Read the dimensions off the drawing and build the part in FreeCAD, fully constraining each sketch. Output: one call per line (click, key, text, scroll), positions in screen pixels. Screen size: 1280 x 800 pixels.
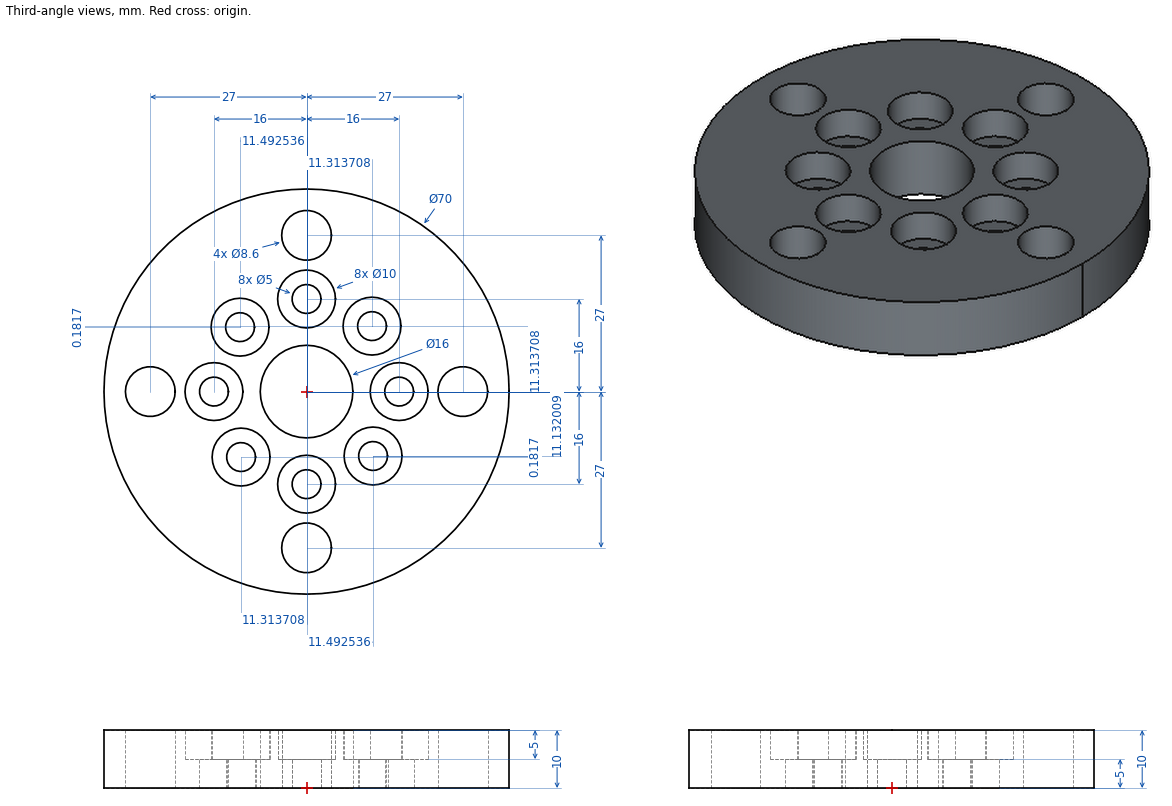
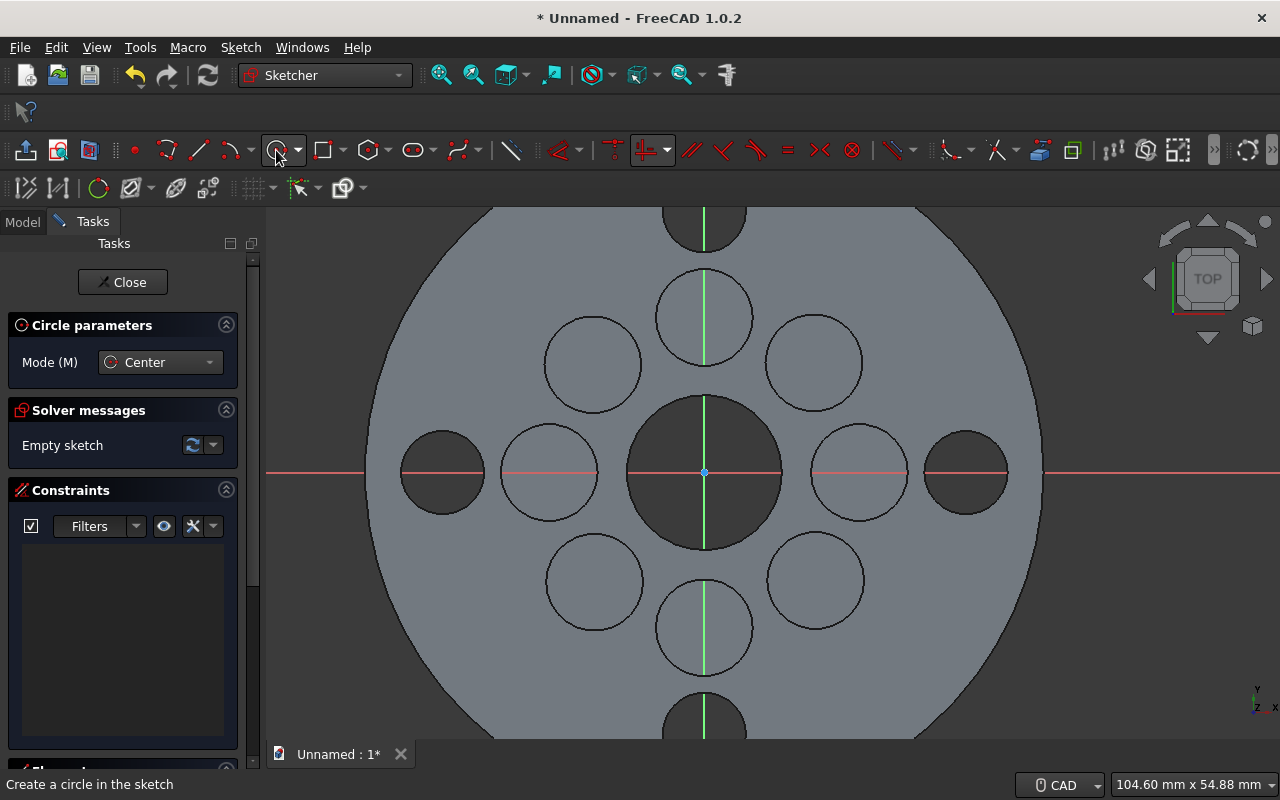
click(704, 317)
move(721, 300)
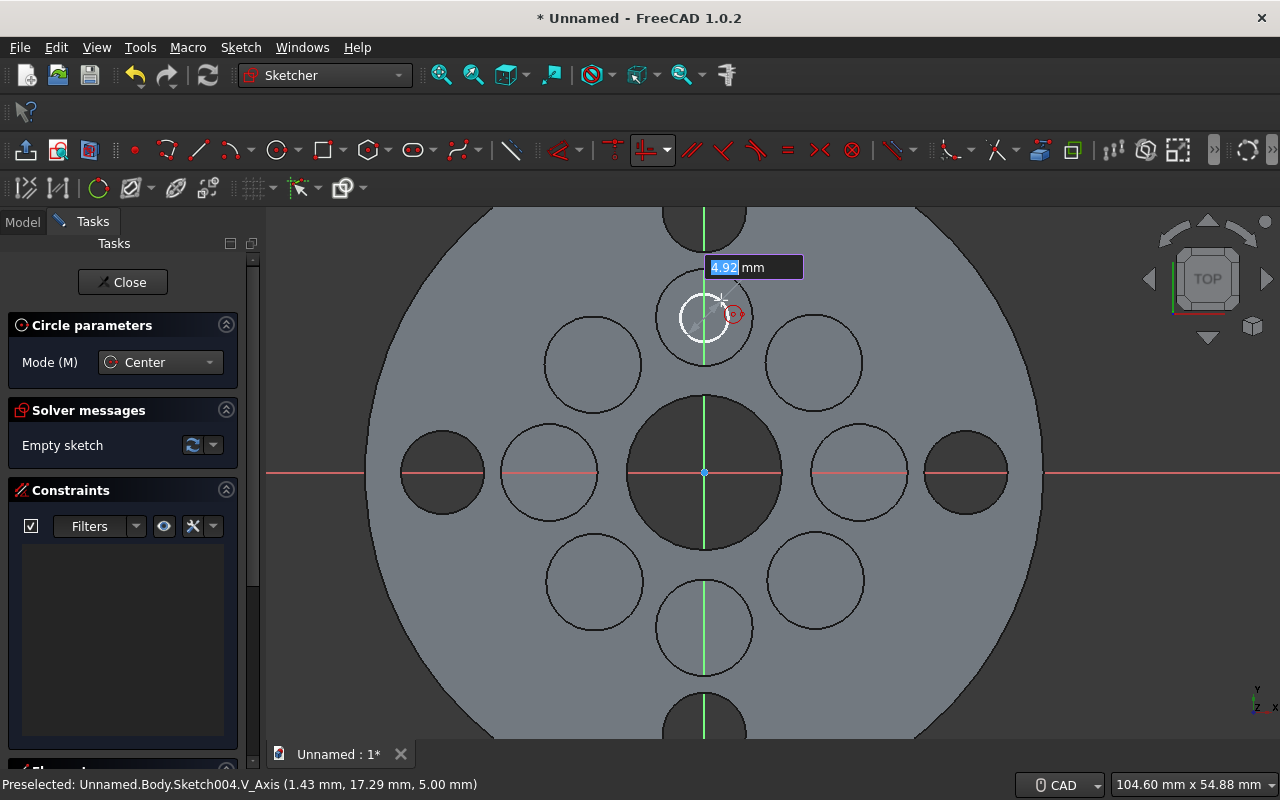
text(5)
key(Return)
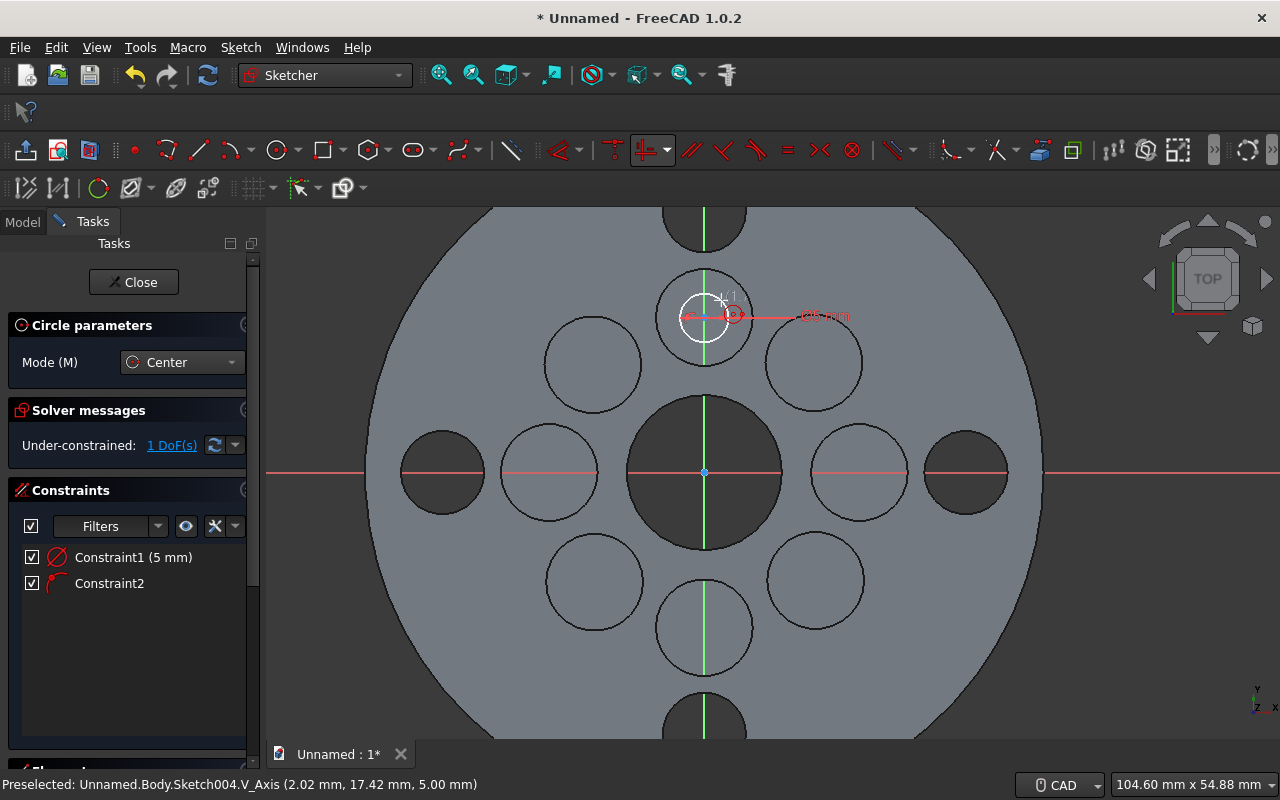
click(814, 363)
move(831, 346)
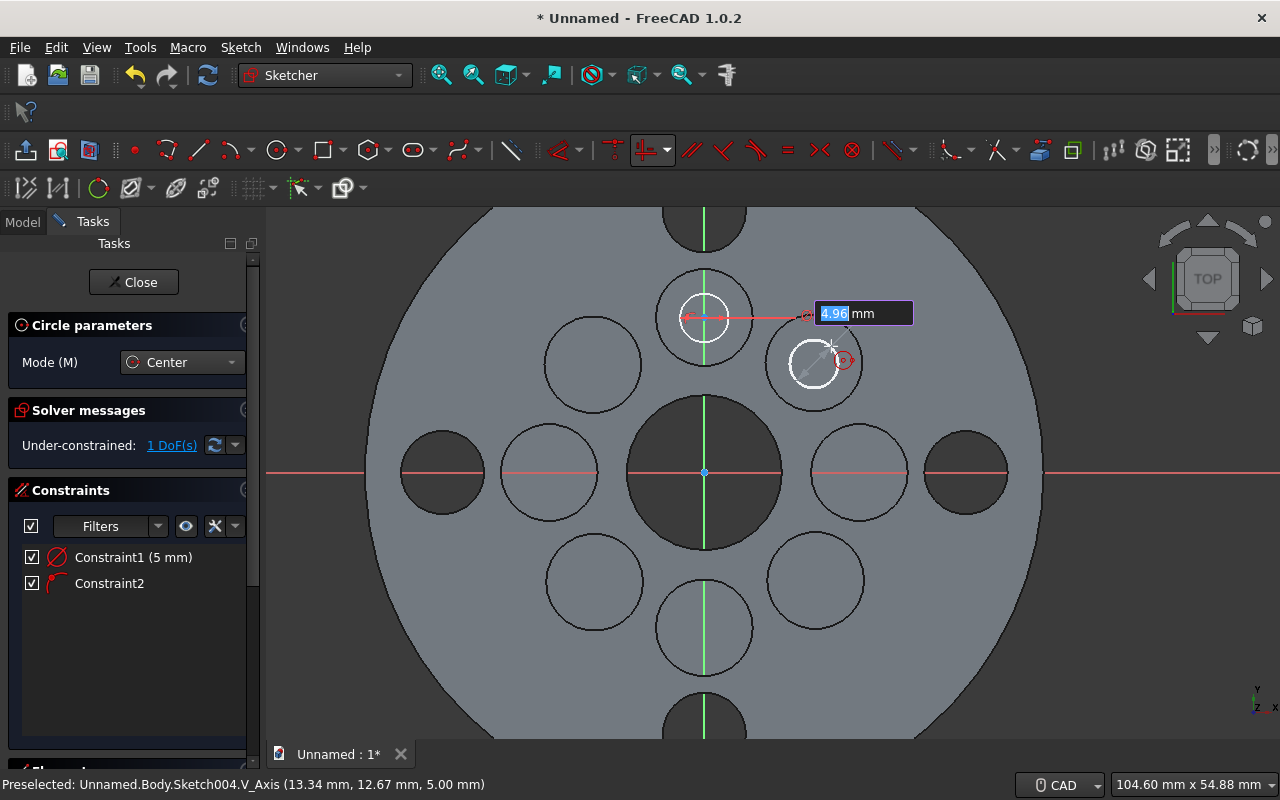
text(5)
key(Return)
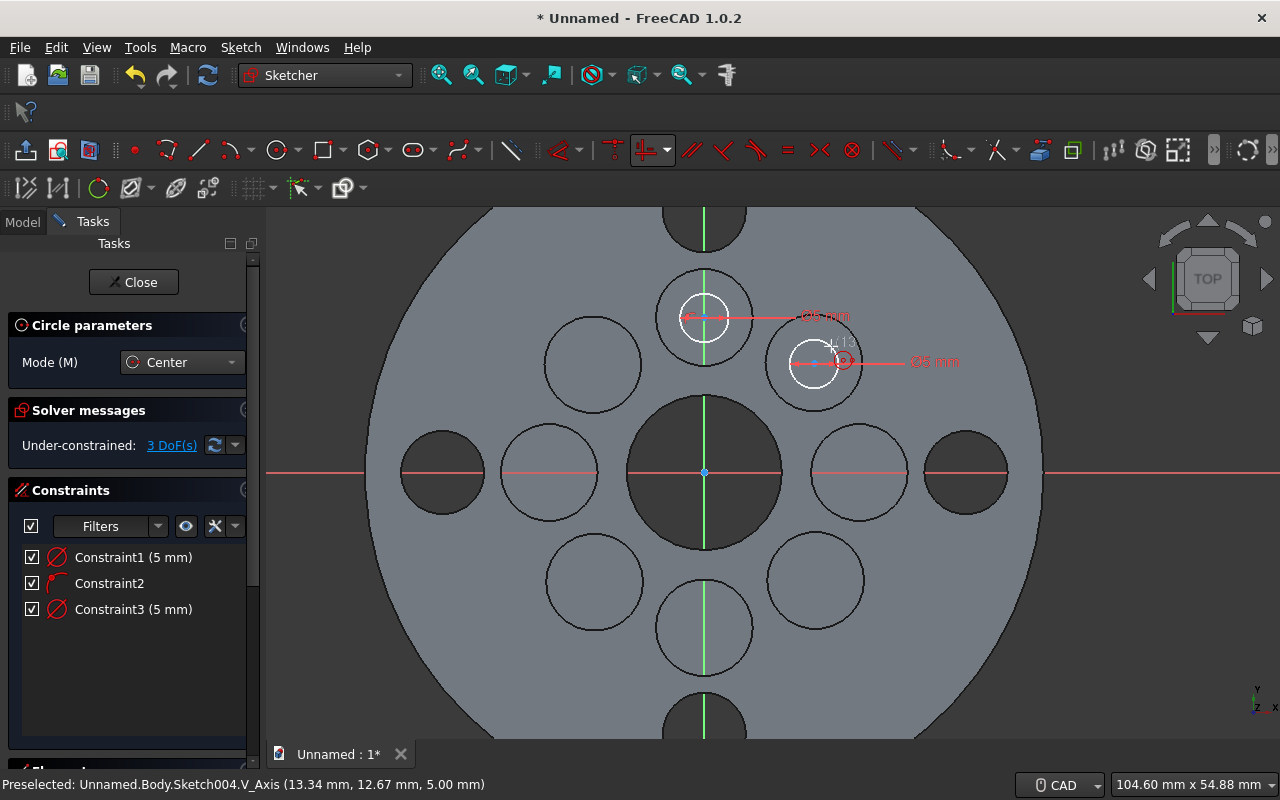
click(859, 473)
move(877, 455)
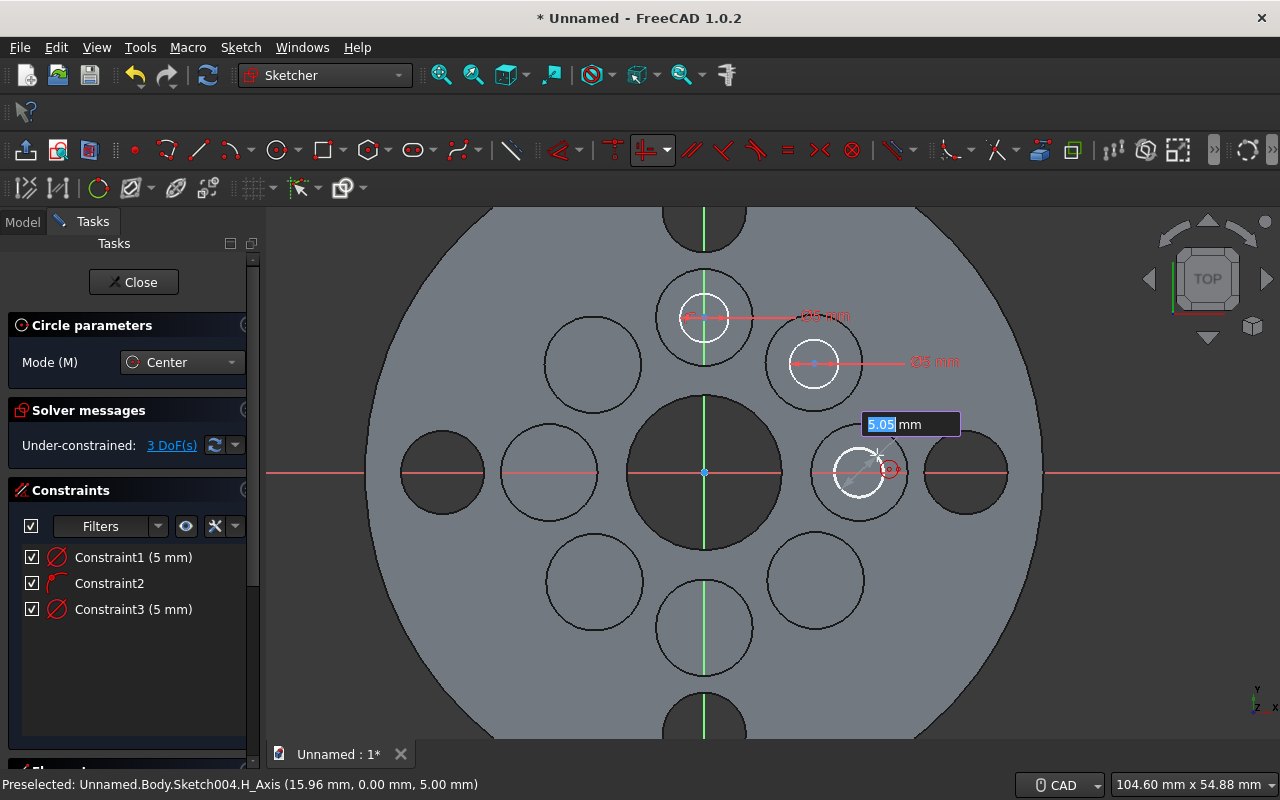
text(5)
key(Return)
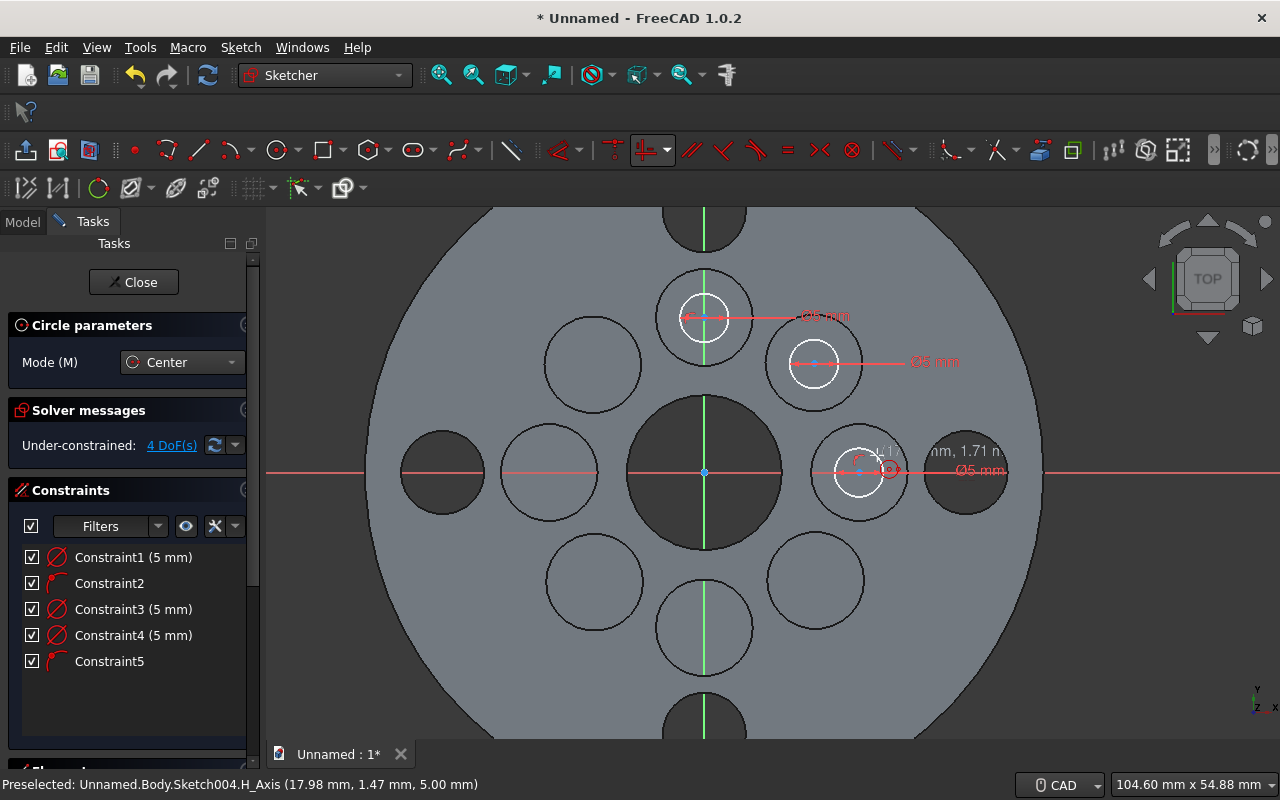
click(816, 580)
move(833, 563)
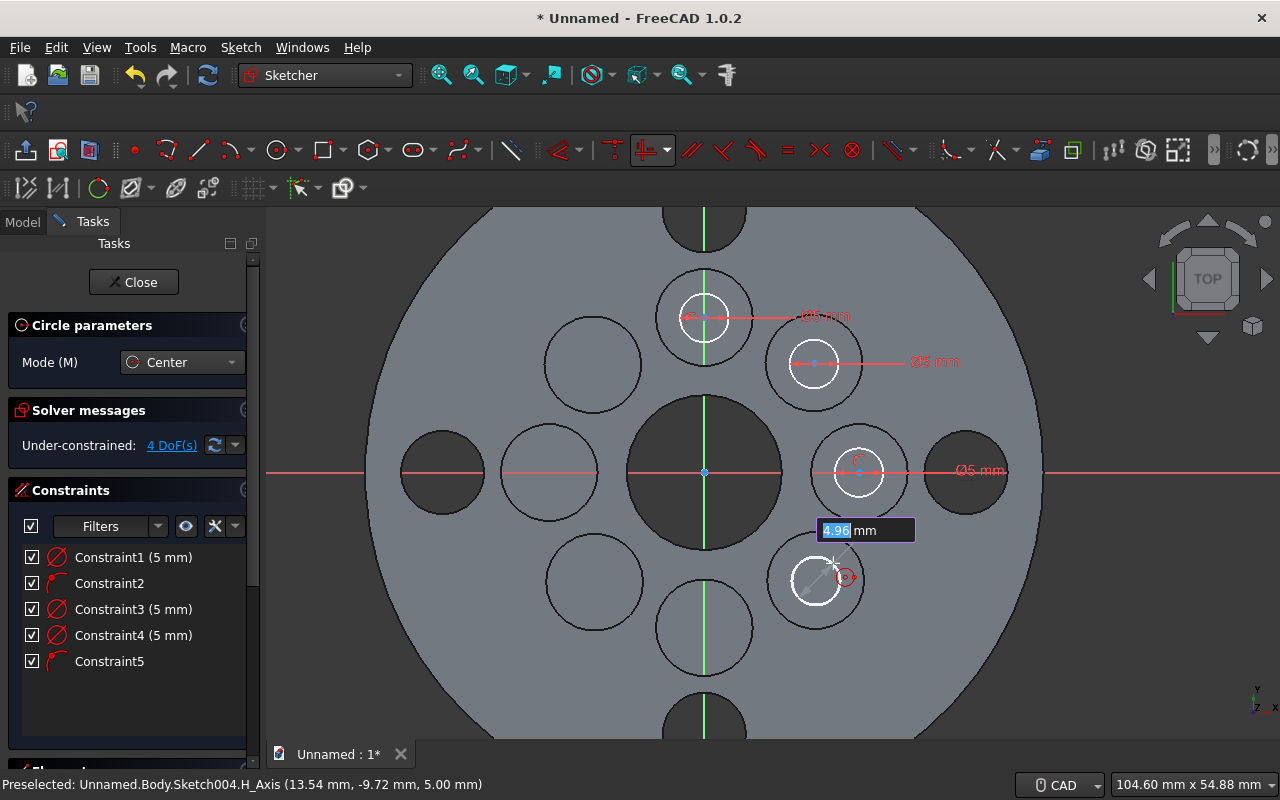
text(5)
key(Return)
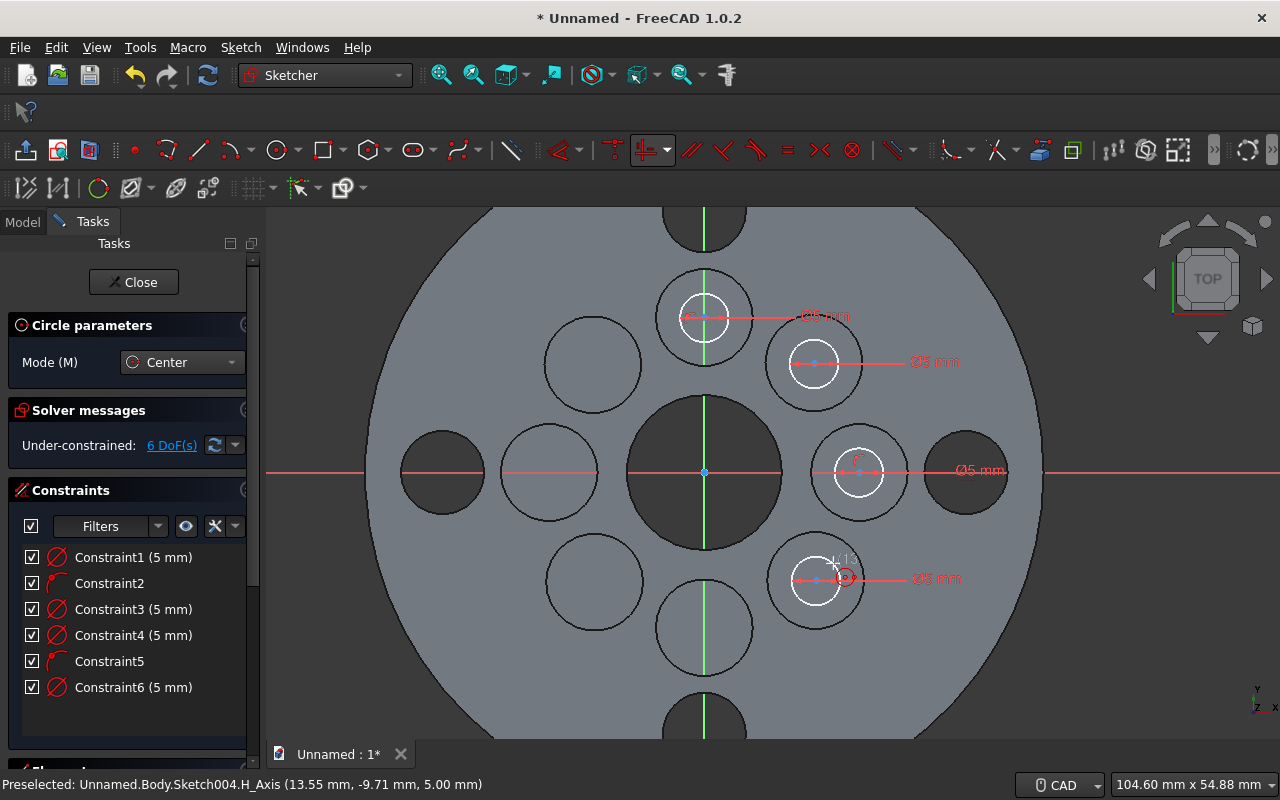
click(704, 628)
move(721, 611)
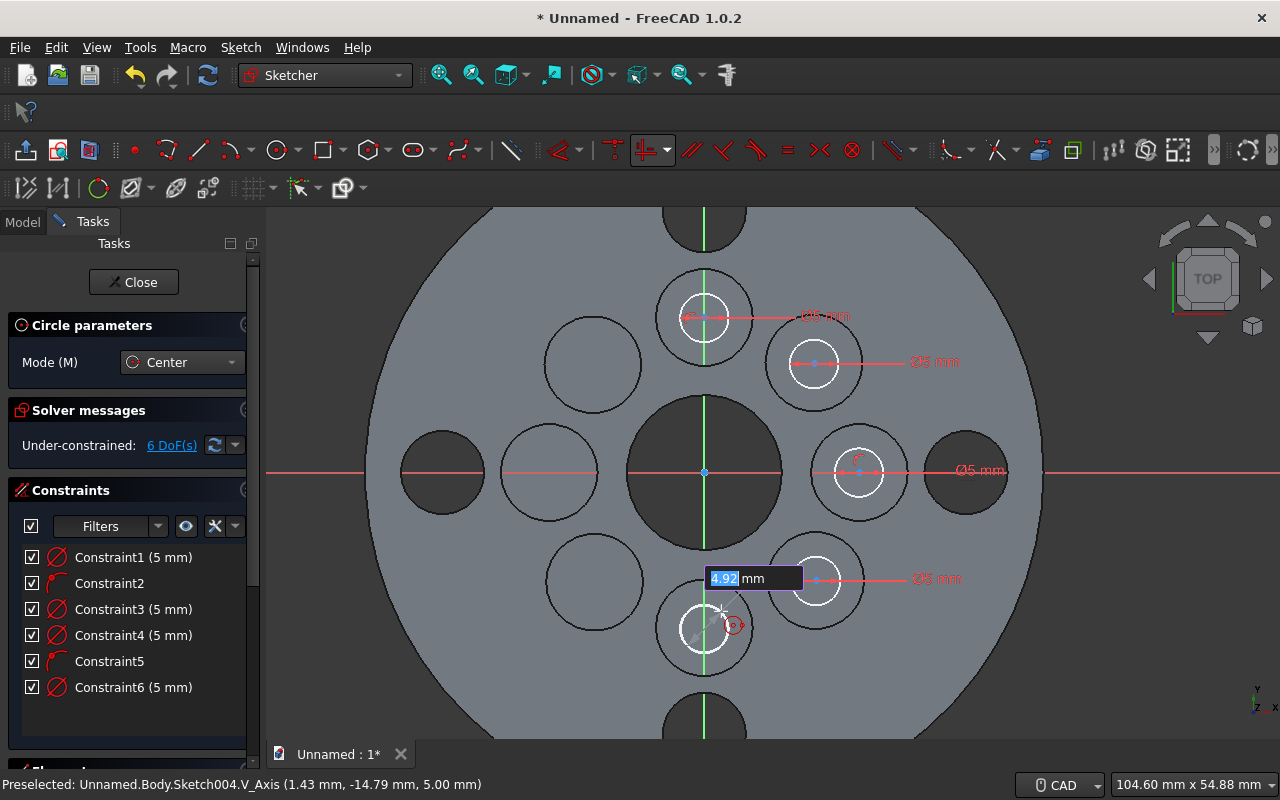
text(5)
key(Return)